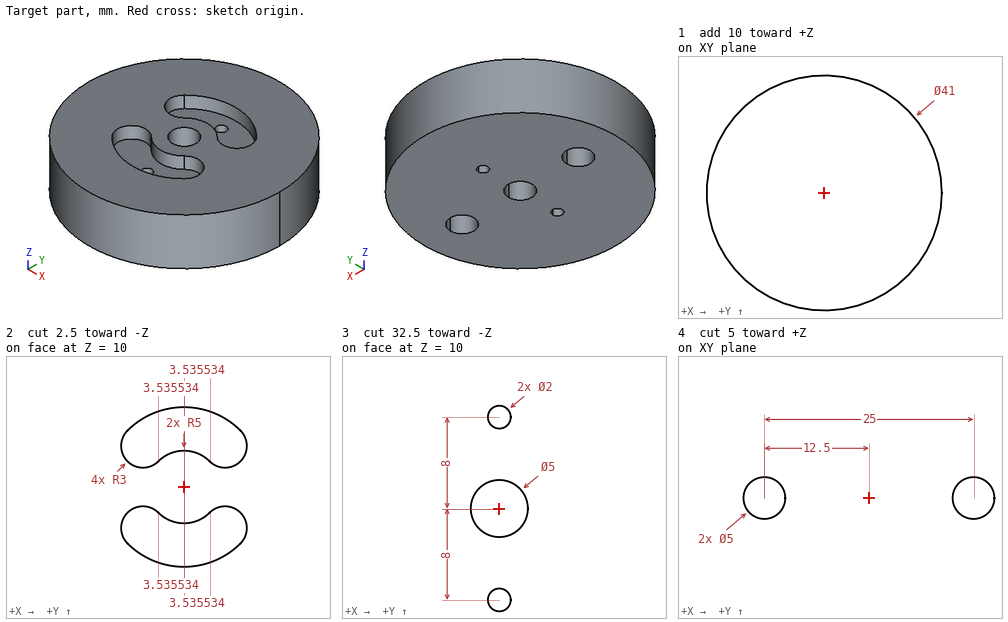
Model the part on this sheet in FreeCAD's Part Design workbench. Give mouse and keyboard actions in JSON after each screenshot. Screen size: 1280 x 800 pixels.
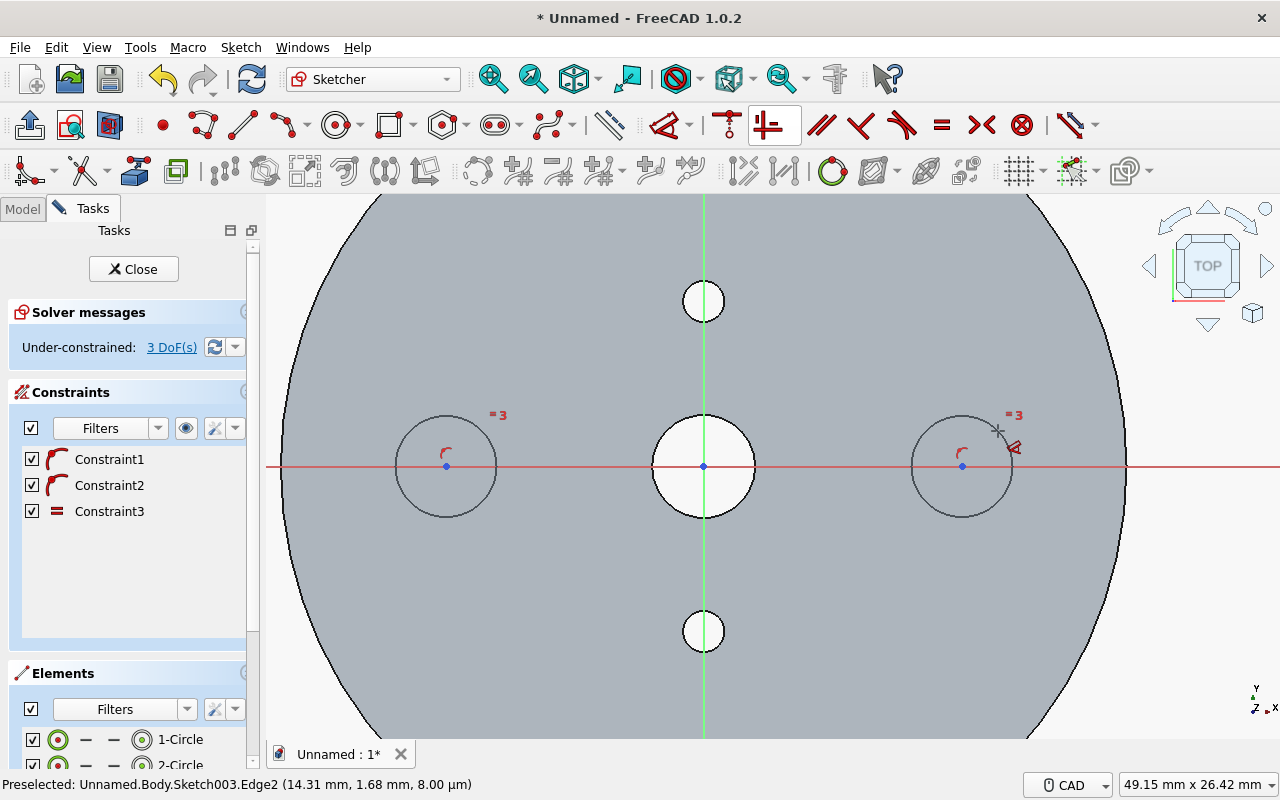
{"action": "left_click", "coordinate": [482, 431]}
{"action": "left_click", "coordinate": [505, 409]}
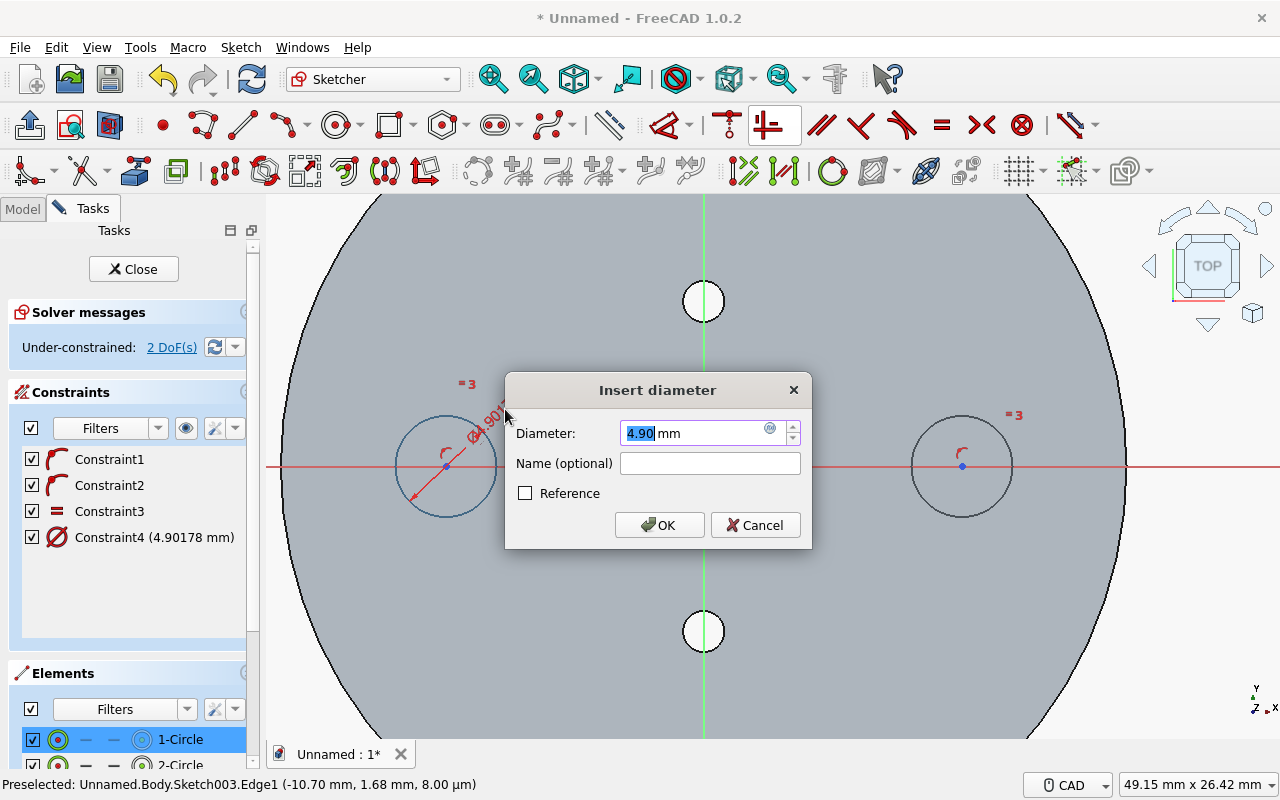
{"action": "type", "text": "5"}
{"action": "key", "text": "Return"}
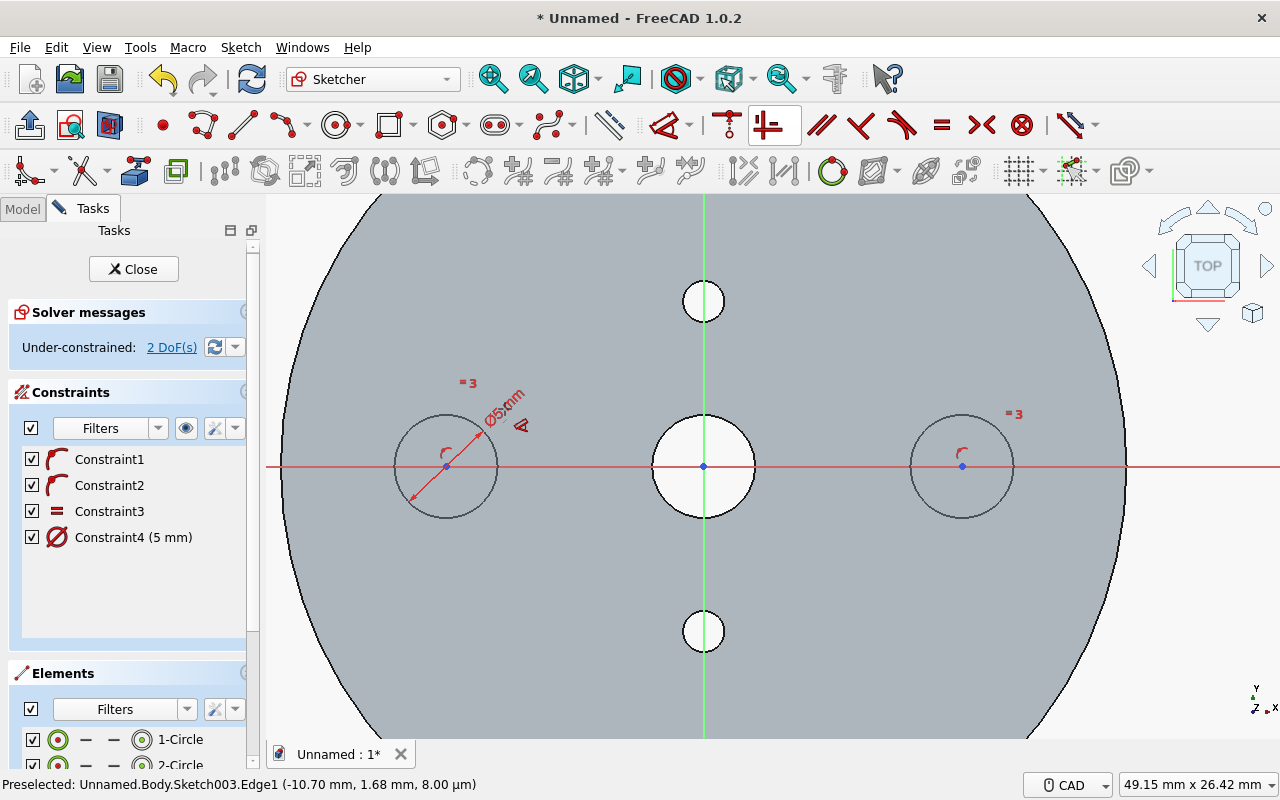
{"action": "left_click", "coordinate": [446, 466]}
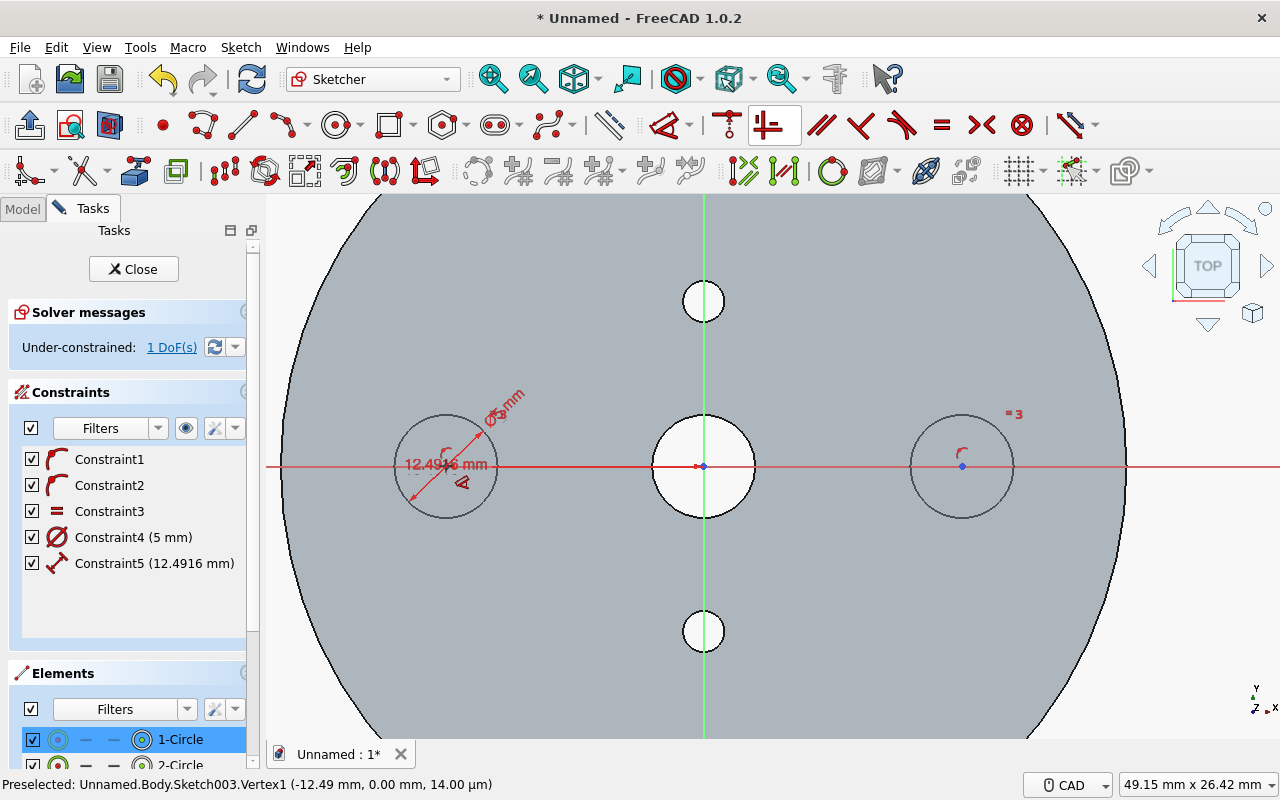
{"action": "left_click", "coordinate": [962, 466]}
{"action": "left_click", "coordinate": [585, 500]}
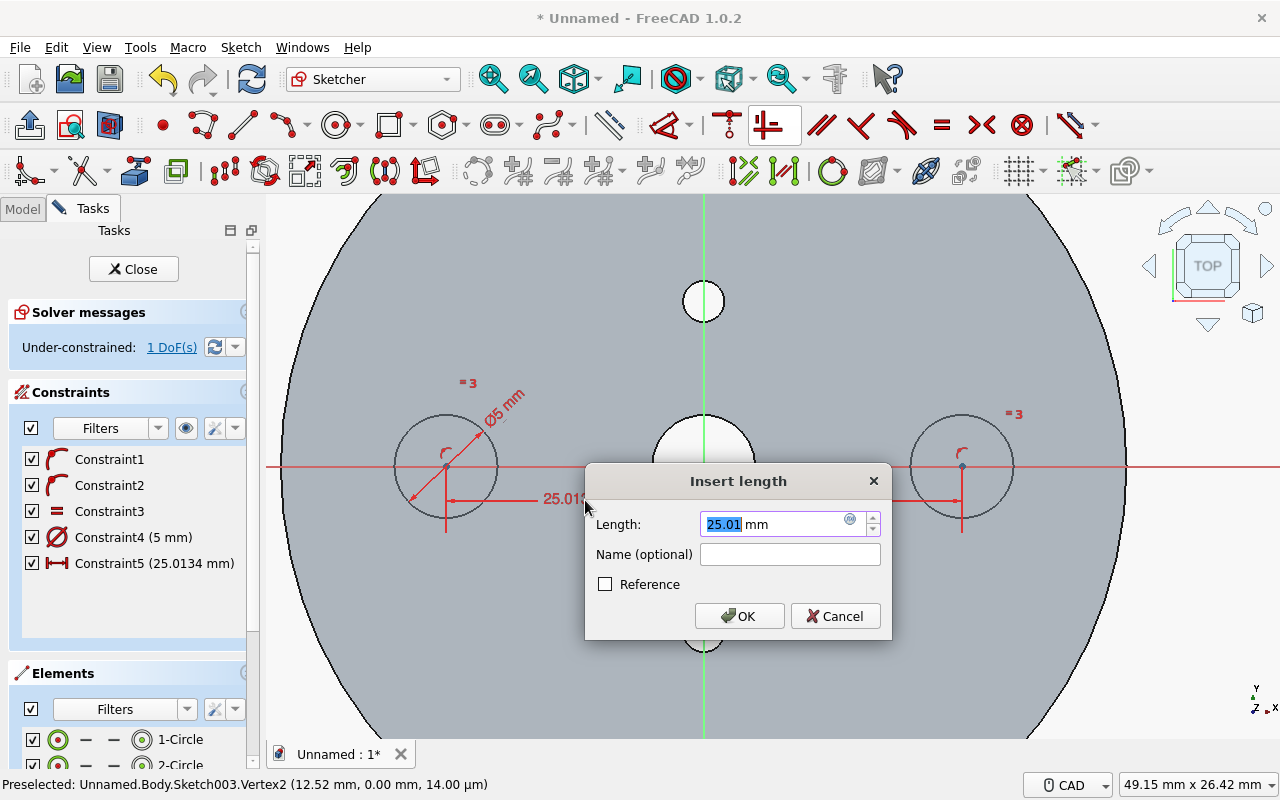
{"action": "type", "text": "25"}
{"action": "key", "text": "Return"}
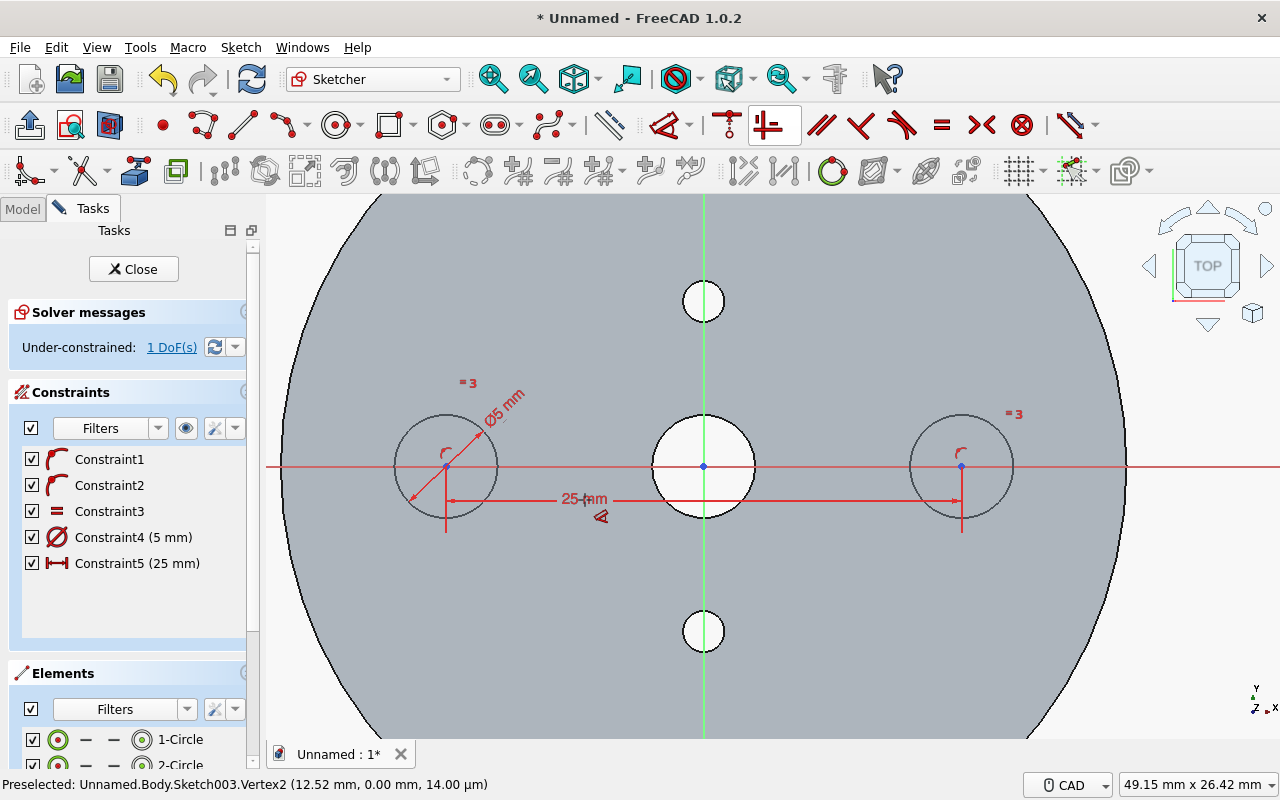
{"action": "left_click", "coordinate": [446, 466]}
{"action": "left_click", "coordinate": [665, 500]}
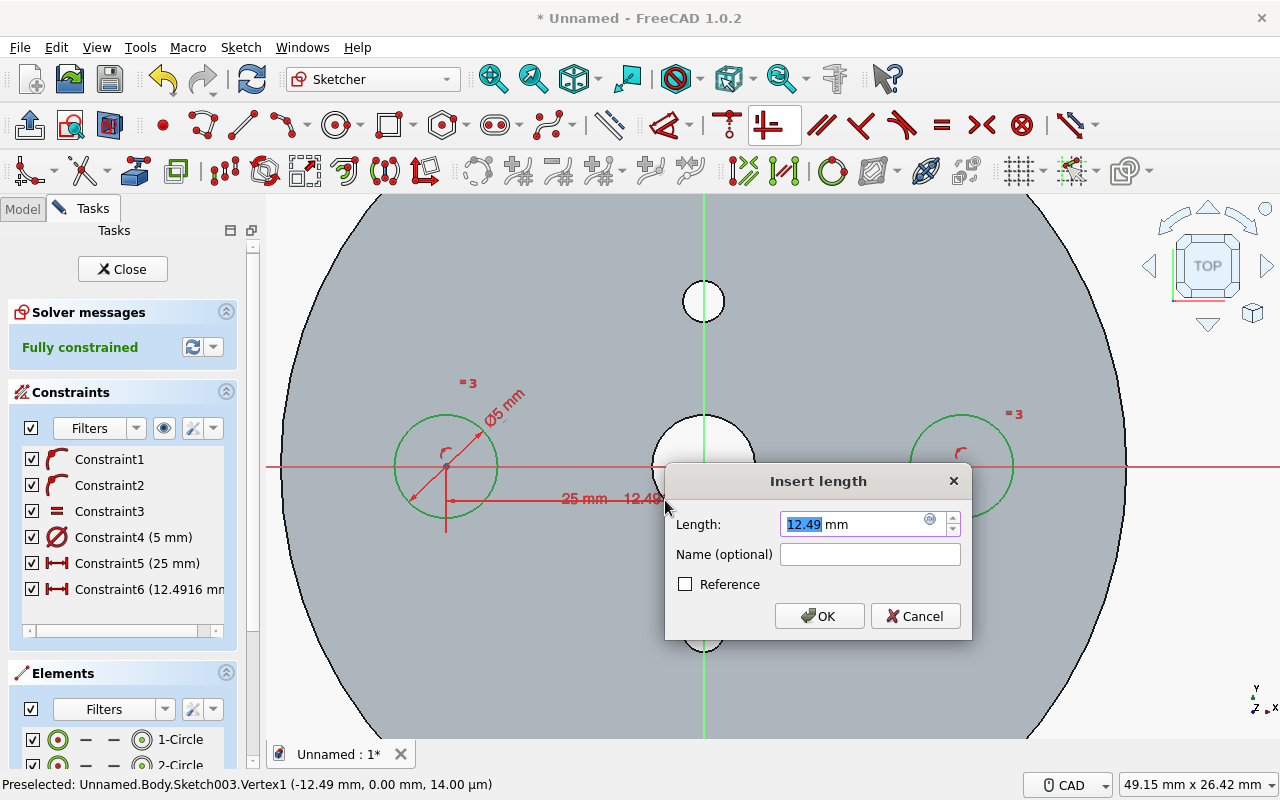
{"action": "type", "text": "12.5"}
{"action": "key", "text": "Return"}
{"action": "key", "text": "Escape"}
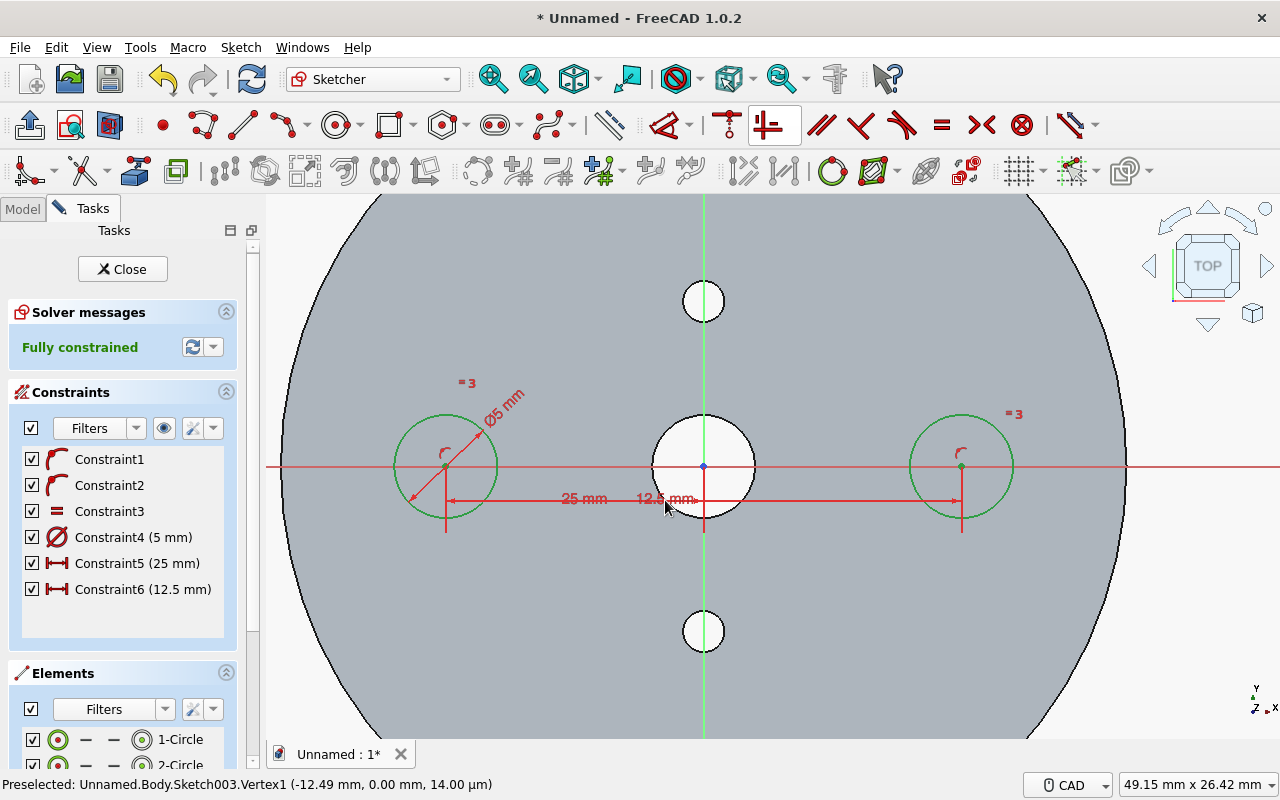
{"action": "left_click", "coordinate": [123, 269]}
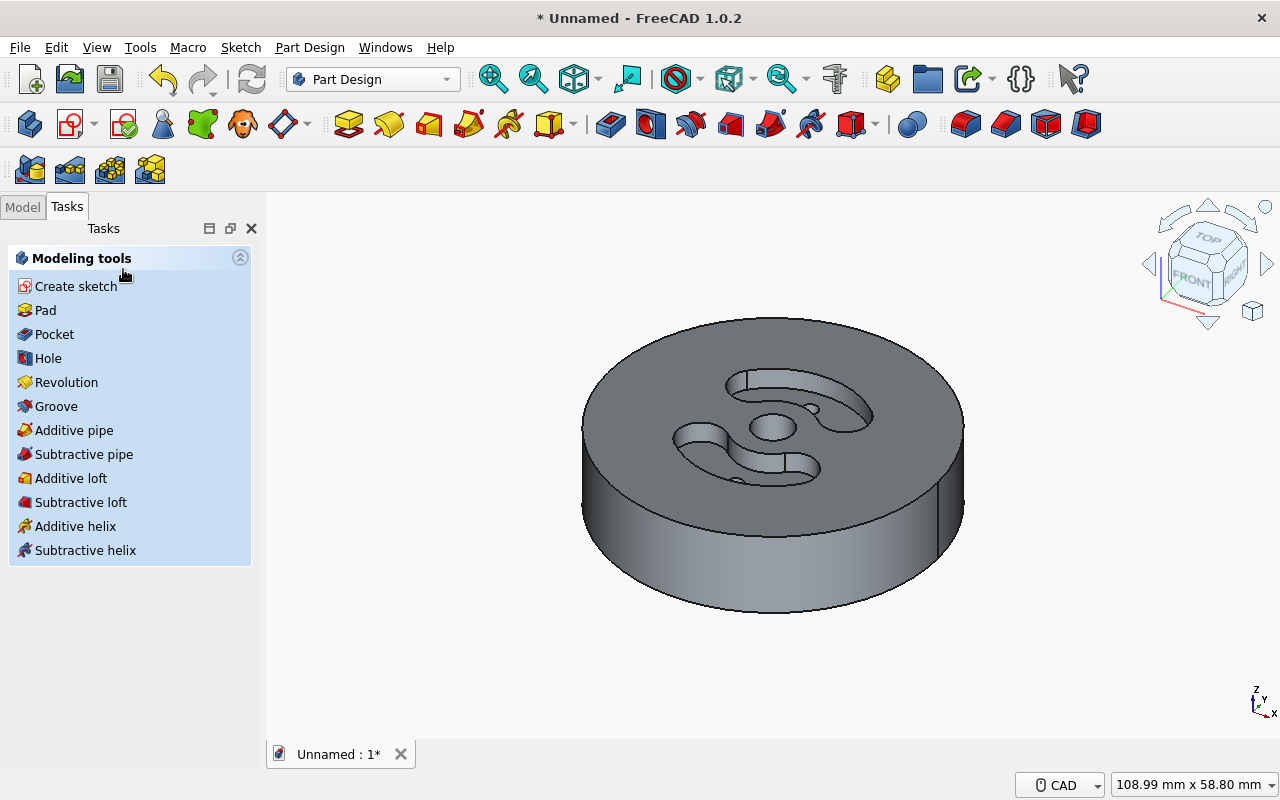
{"action": "left_click", "coordinate": [612, 124]}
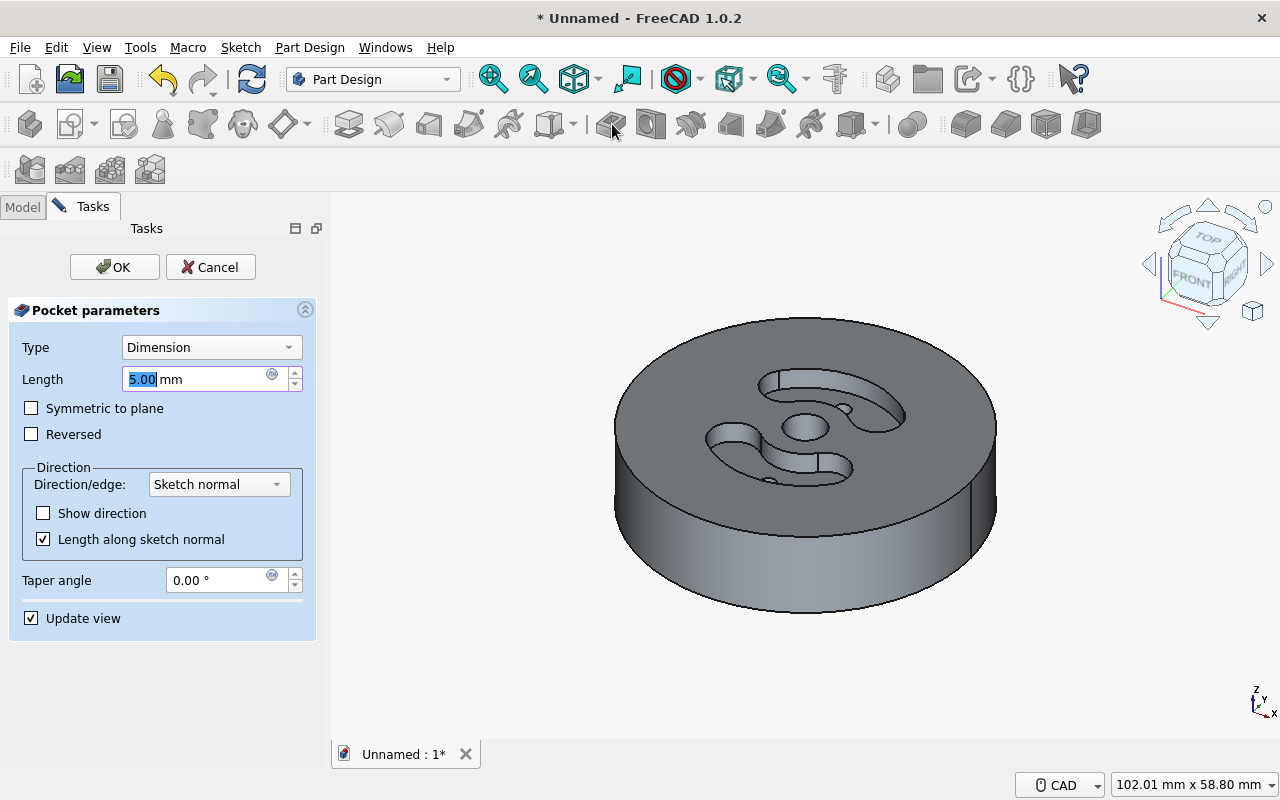
{"action": "type", "text": "5"}
{"action": "key", "text": "Tab"}